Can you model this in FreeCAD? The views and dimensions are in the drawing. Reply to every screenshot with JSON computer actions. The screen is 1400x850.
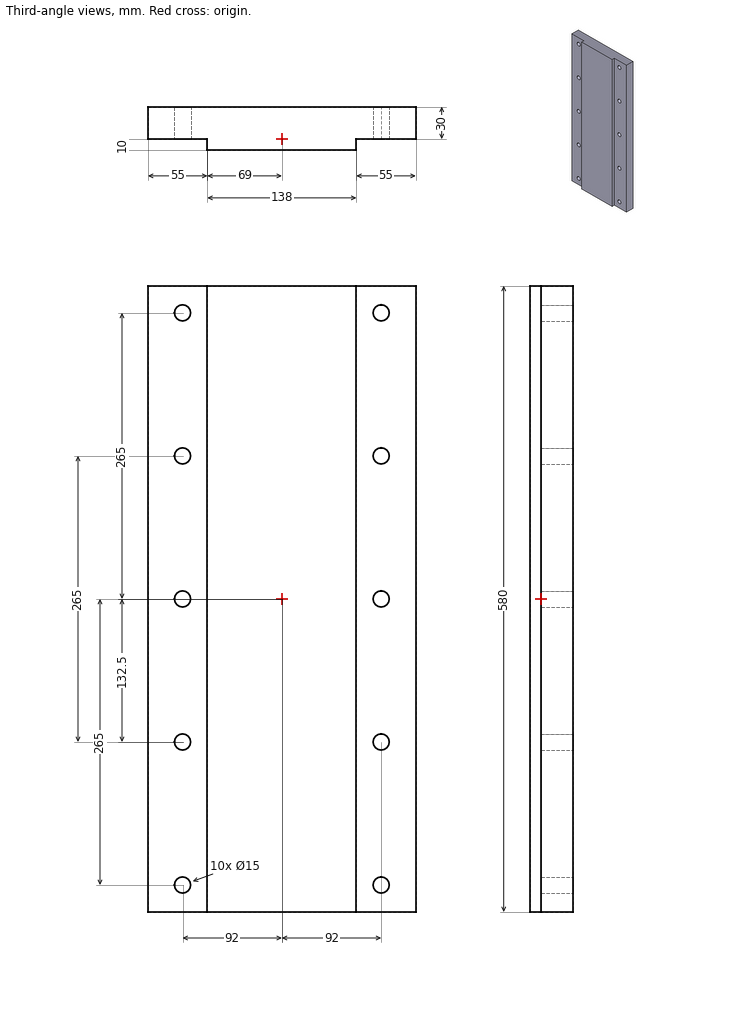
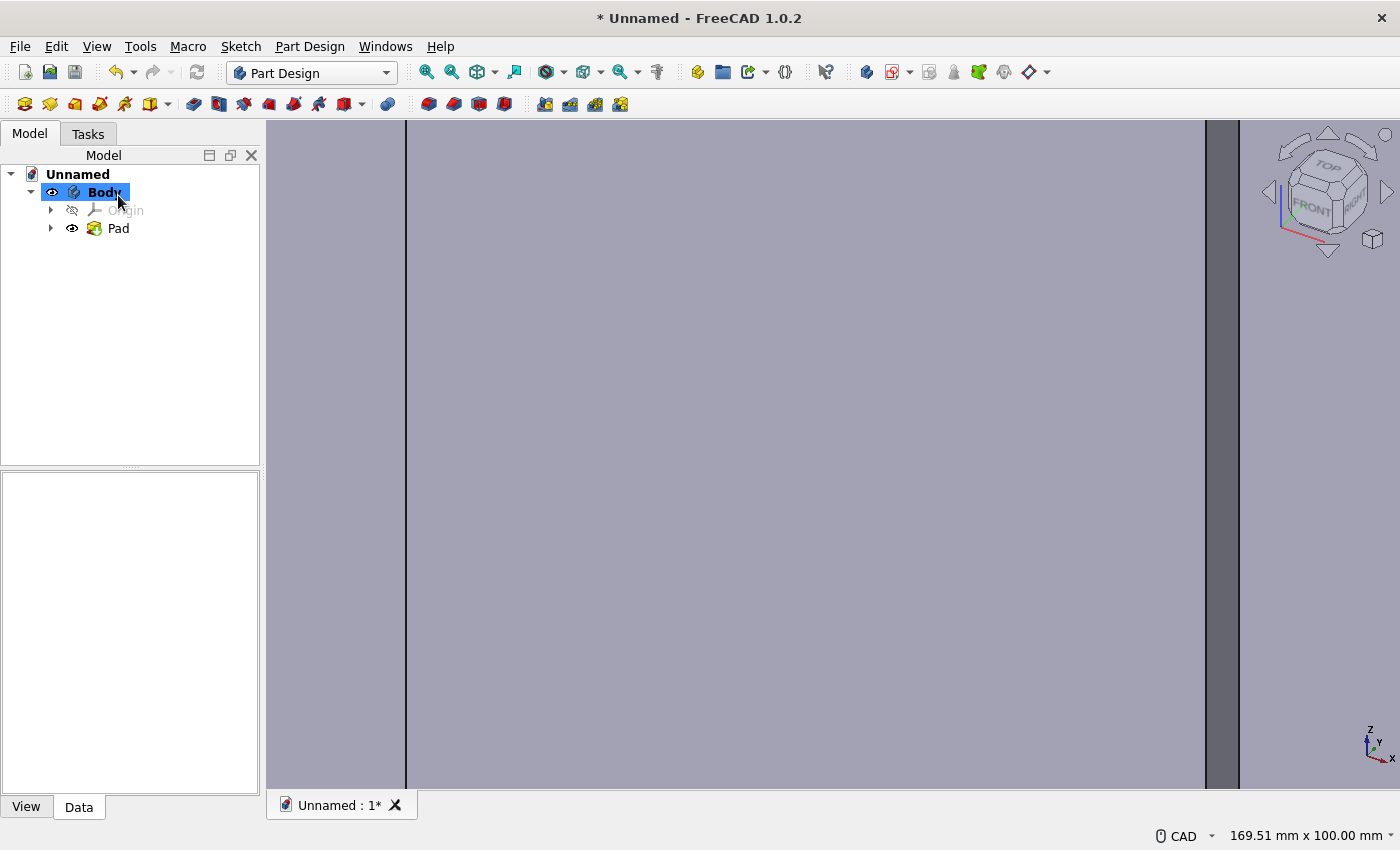
{"action": "left_click", "coordinate": [427, 72]}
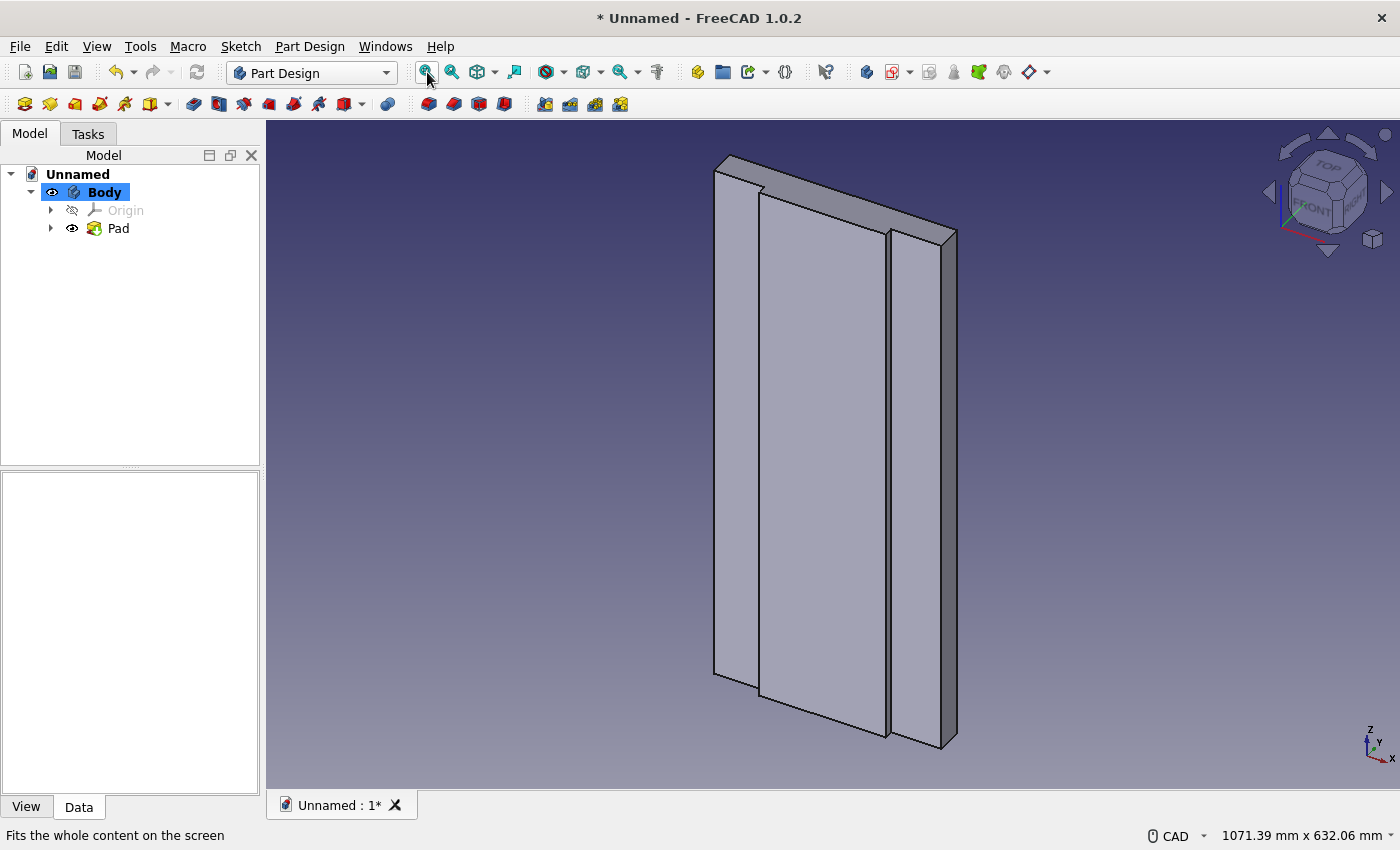
{"action": "key", "text": "4"}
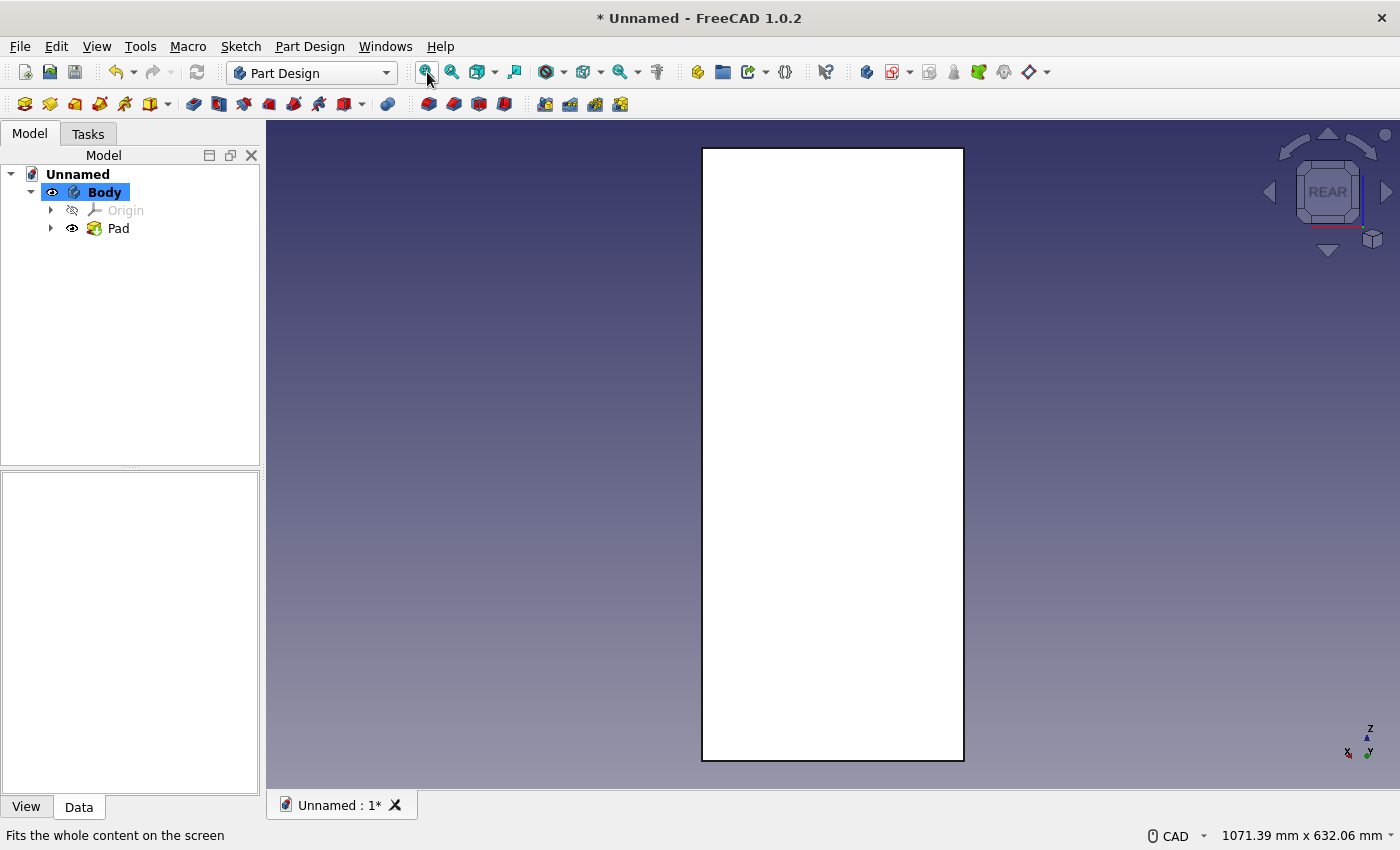
{"action": "left_click", "coordinate": [833, 278]}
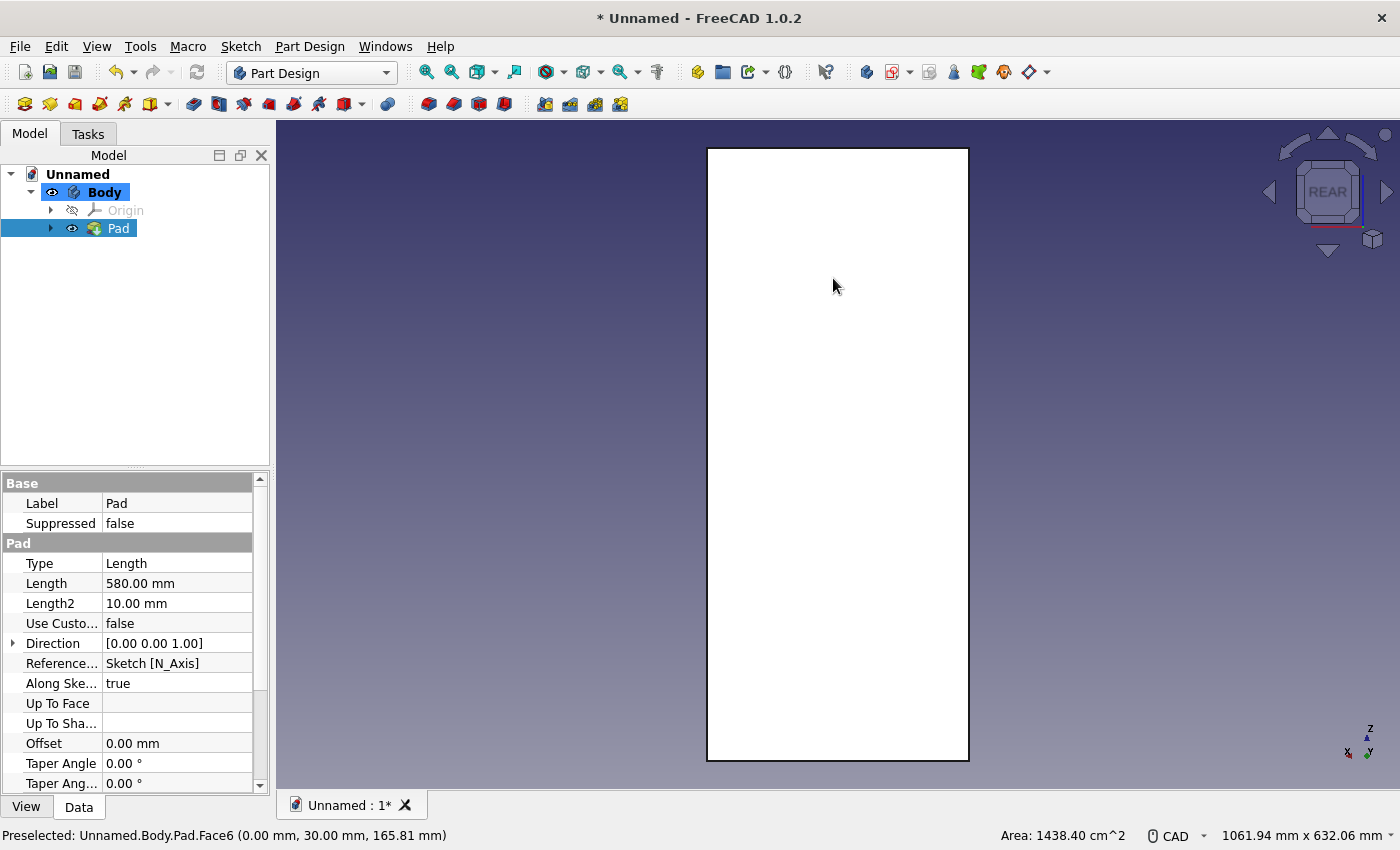
{"action": "left_click", "coordinate": [892, 72]}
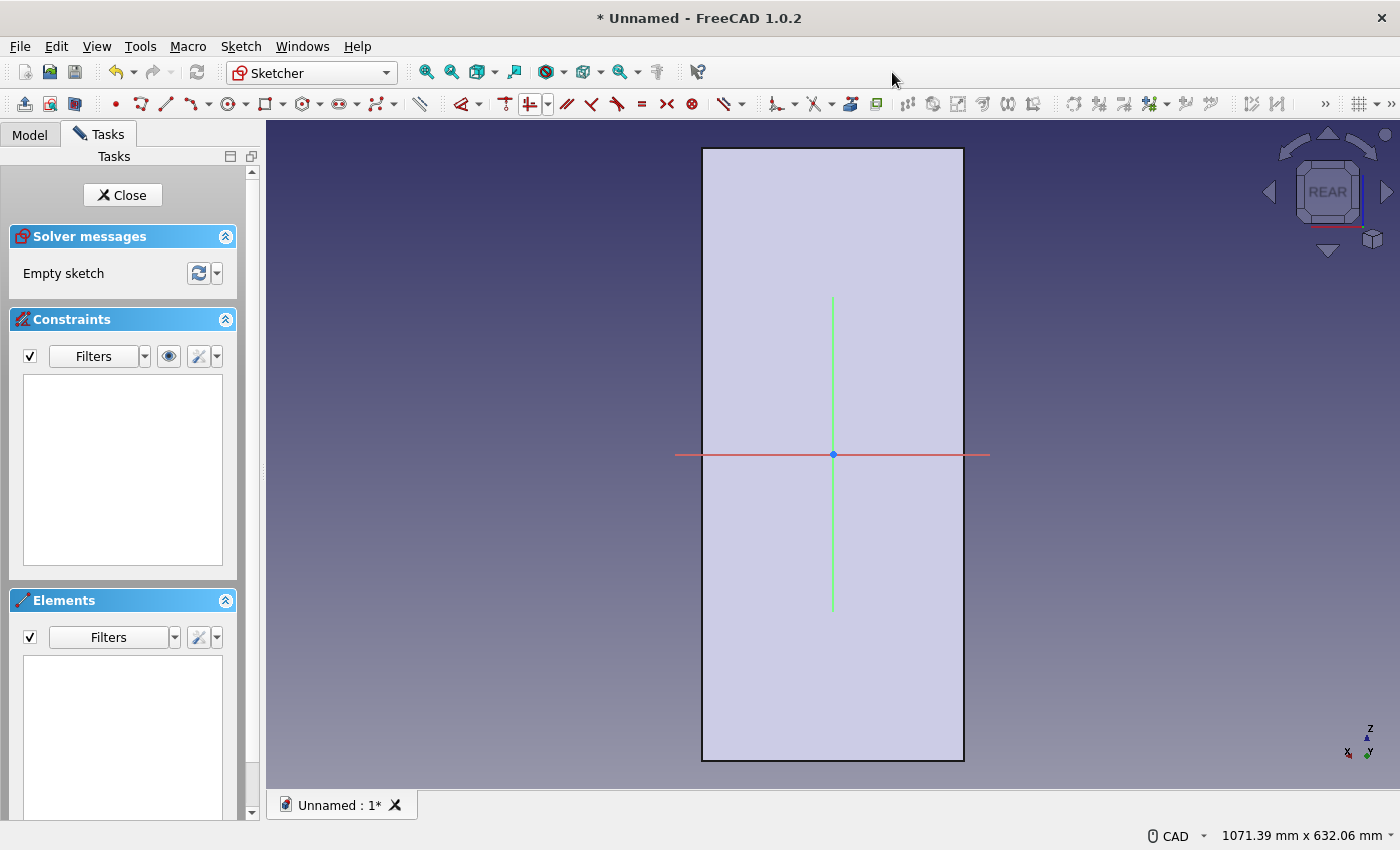
{"action": "scroll", "coordinate": [455, 454], "scroll_direction": "down", "scroll_amount": 1}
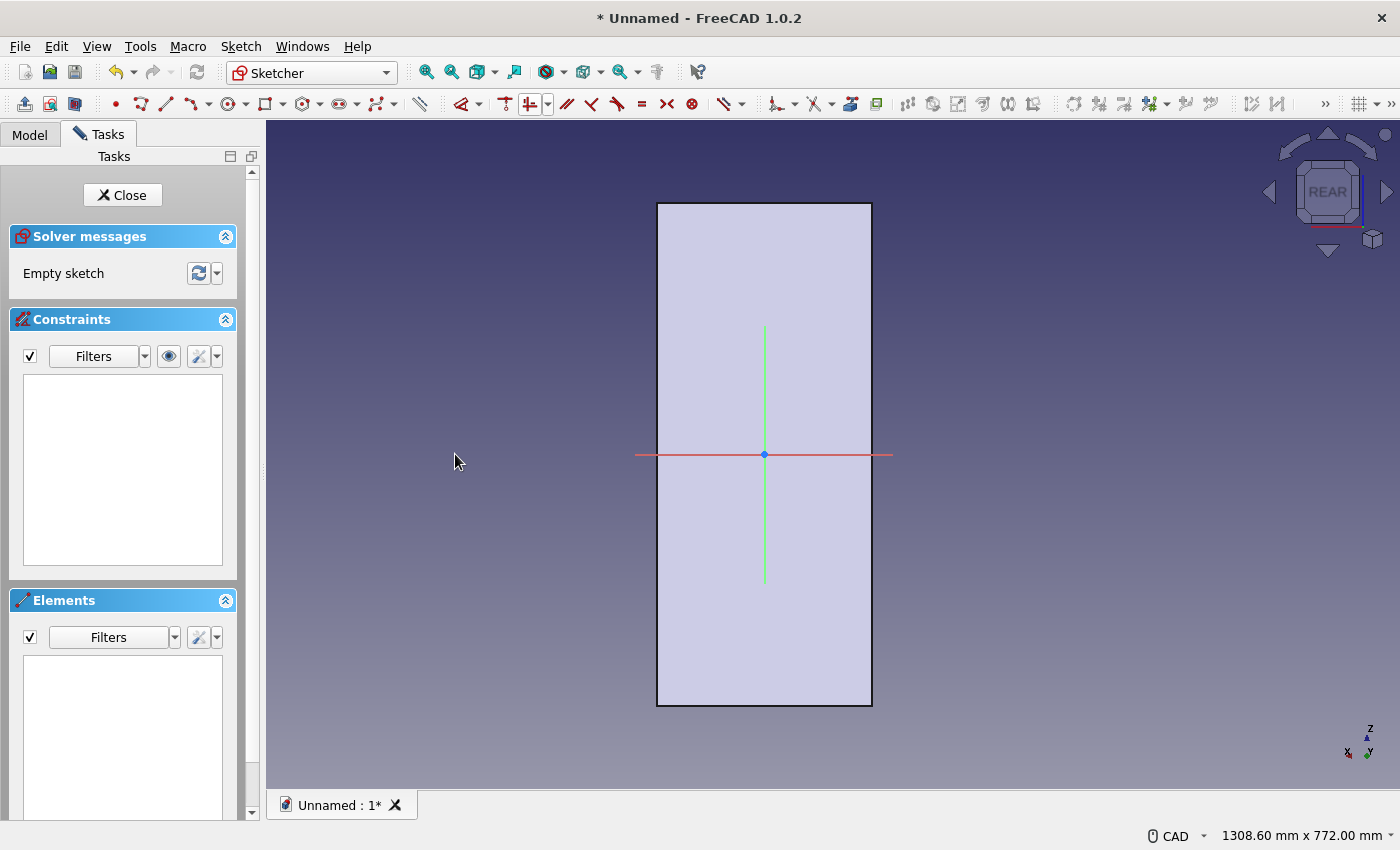
{"action": "key", "text": "g c"}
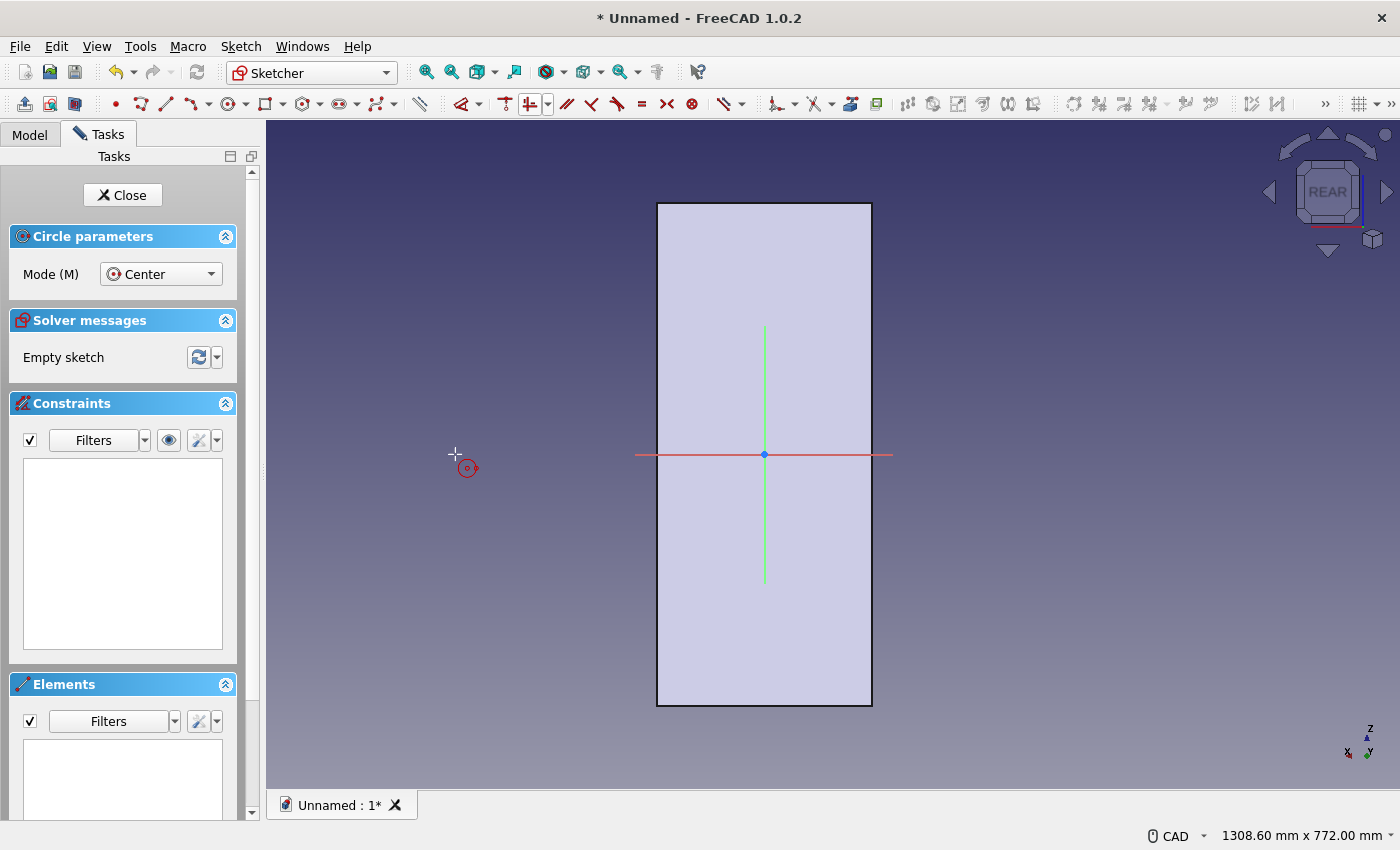
{"action": "scroll", "coordinate": [844, 684], "scroll_direction": "up", "scroll_amount": 7}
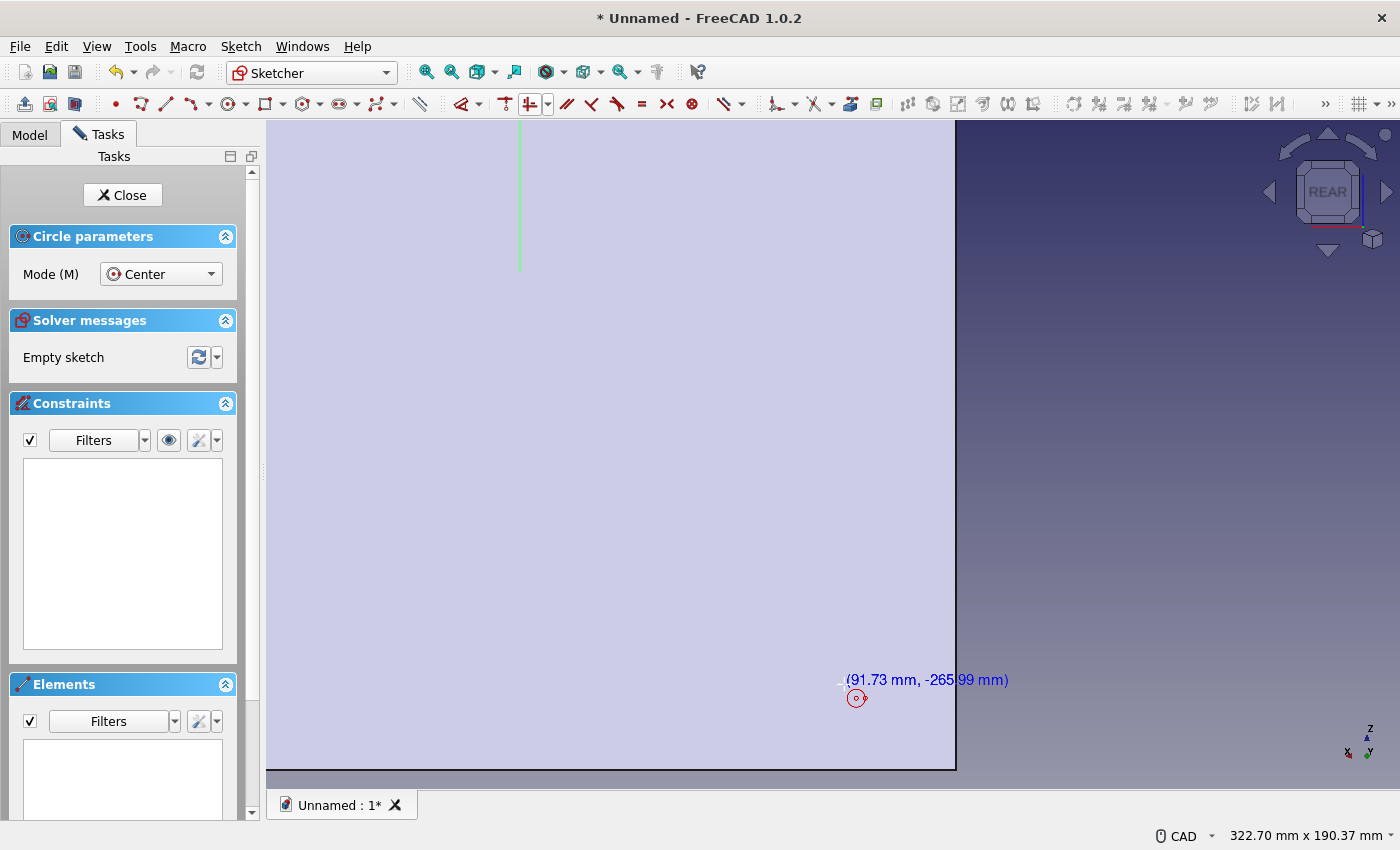
{"action": "scroll", "coordinate": [844, 685], "scroll_direction": "down", "scroll_amount": 7}